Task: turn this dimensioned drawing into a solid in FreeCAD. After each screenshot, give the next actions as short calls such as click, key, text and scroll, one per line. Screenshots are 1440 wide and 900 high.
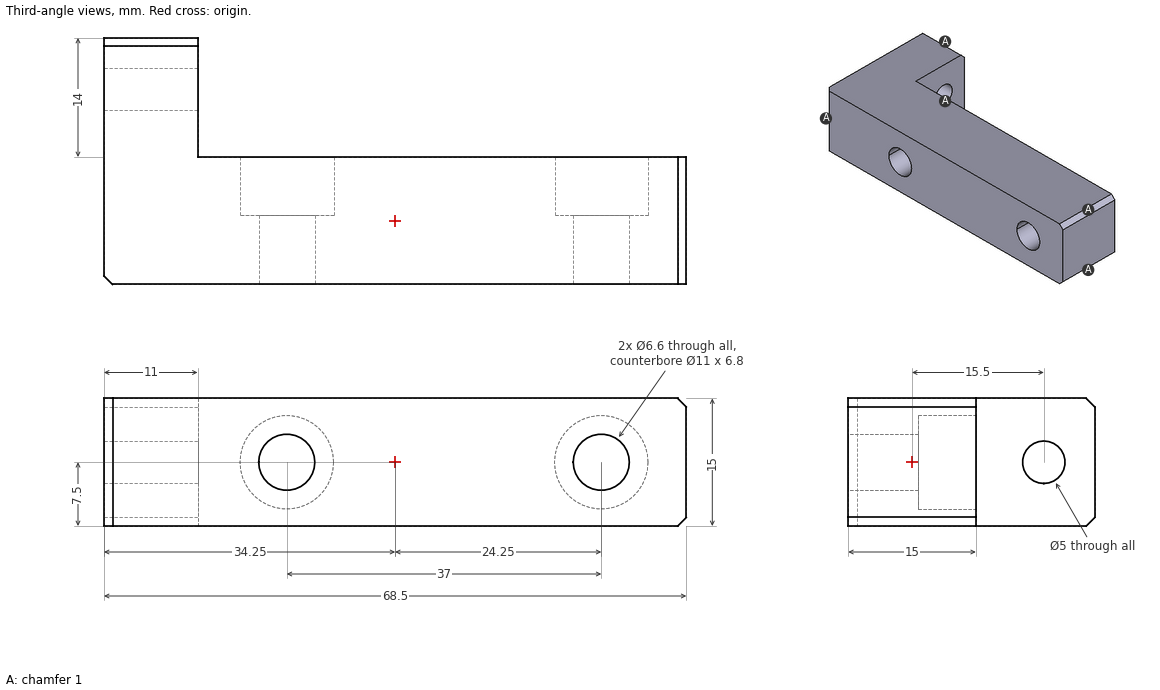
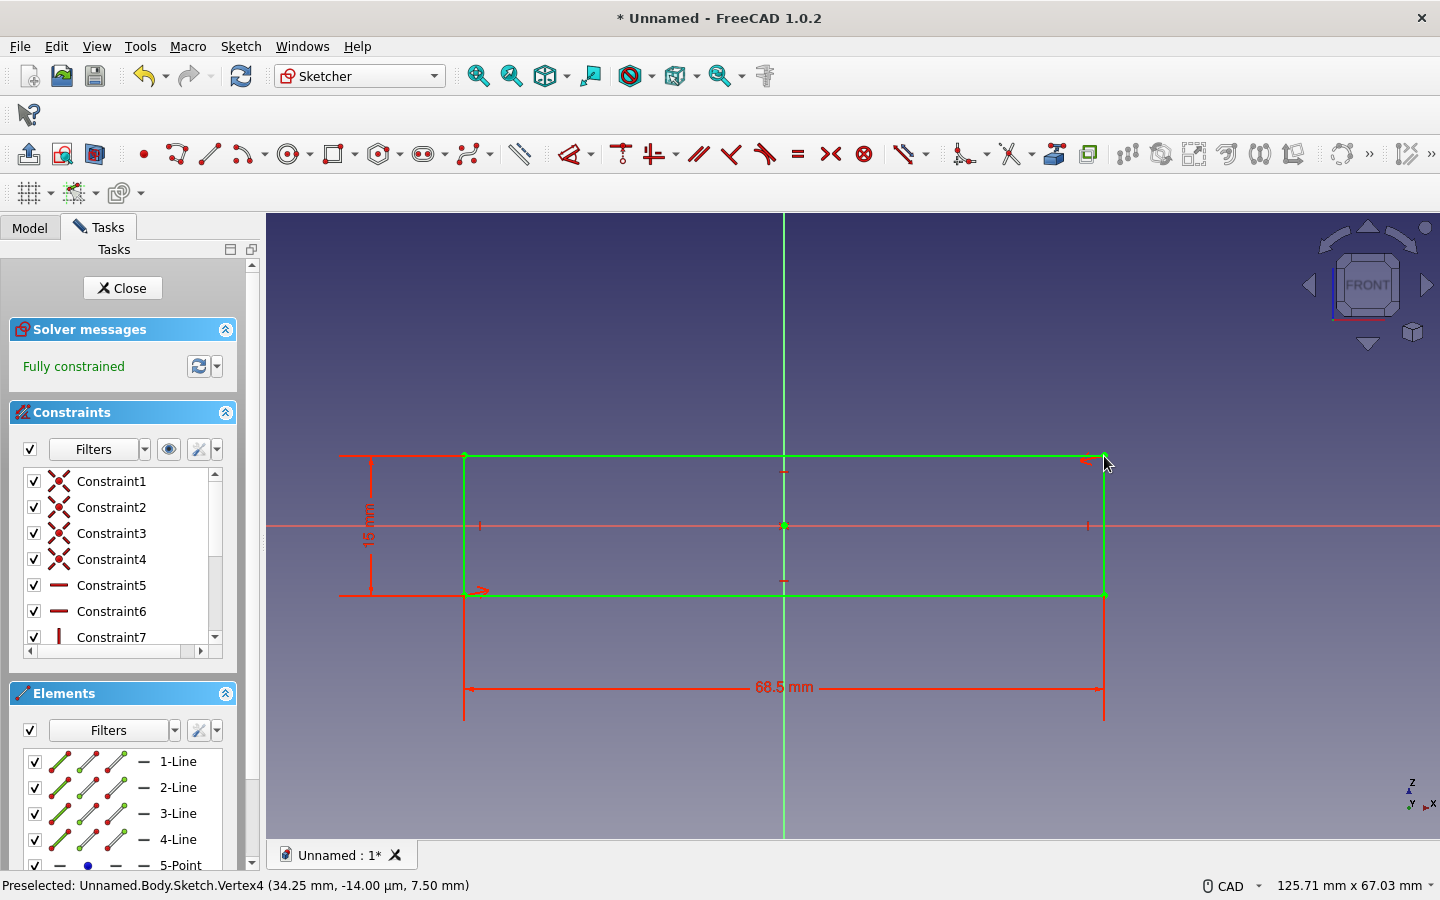
click(123, 288)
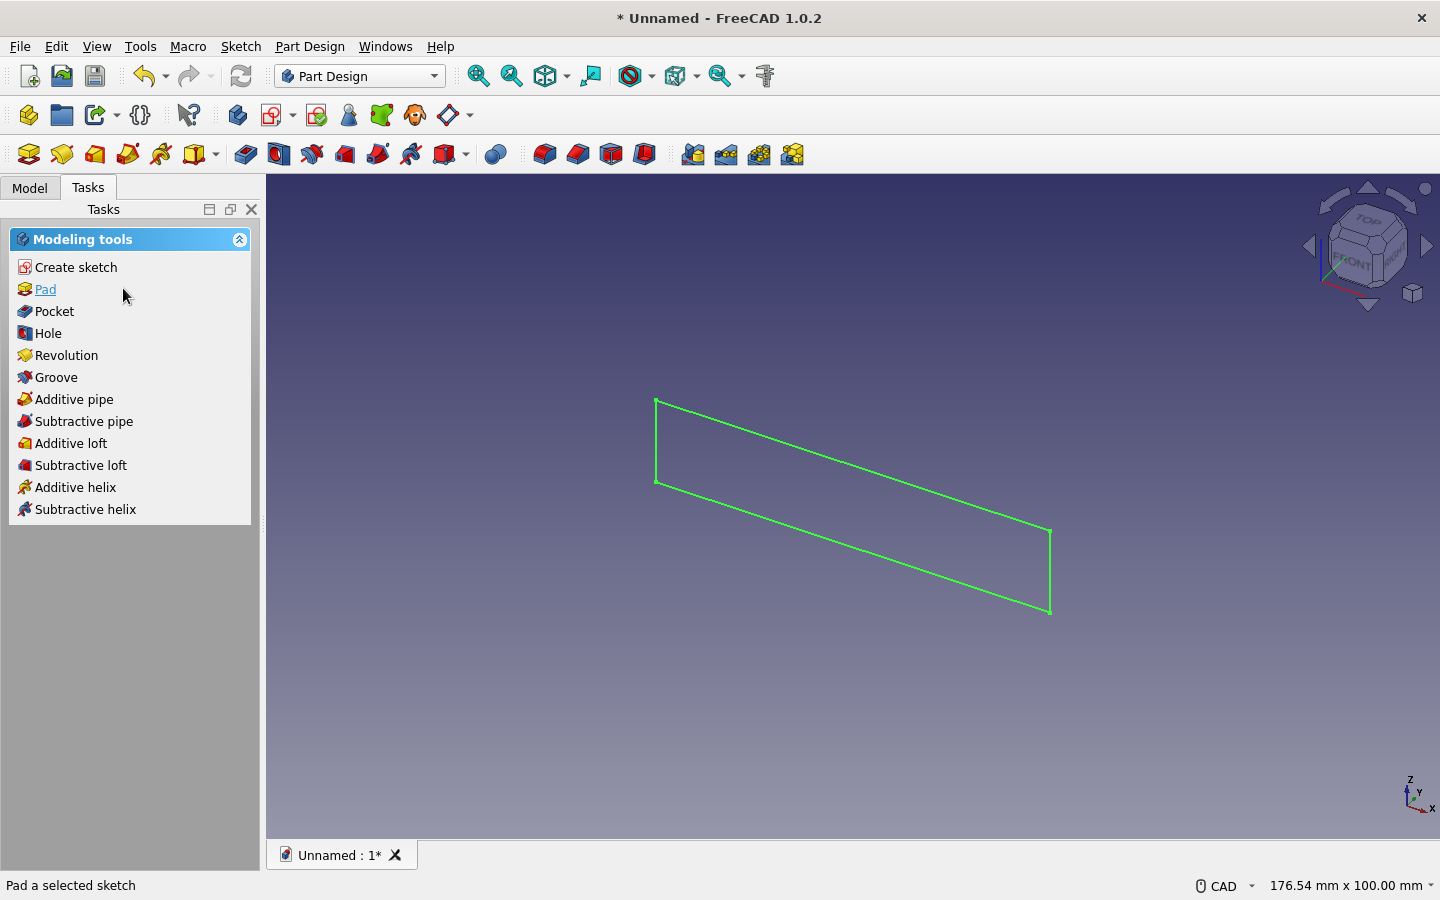
click(29, 154)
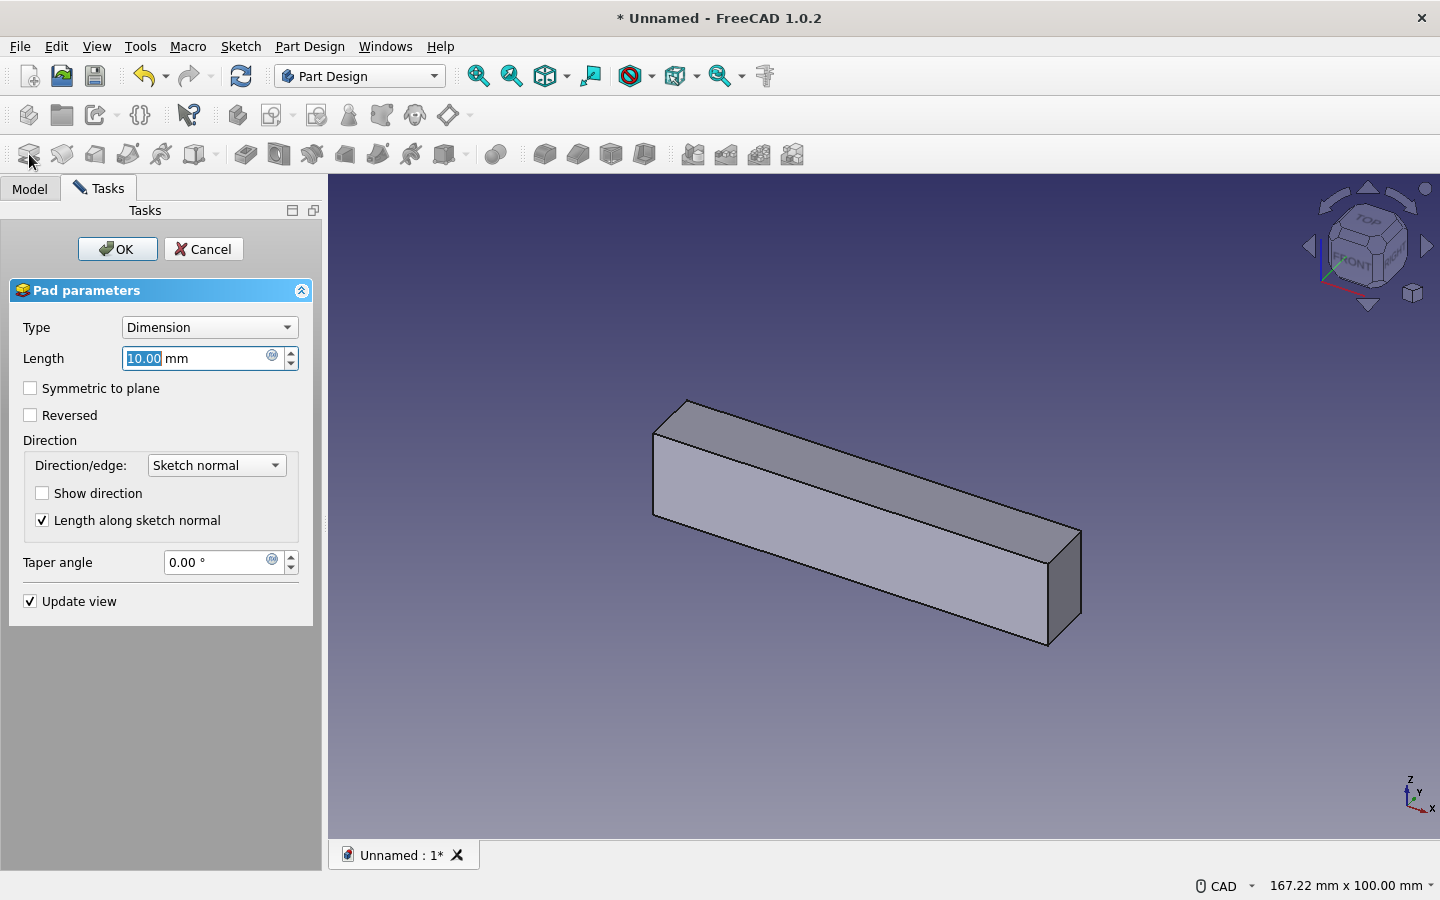
text(15)
key(Tab)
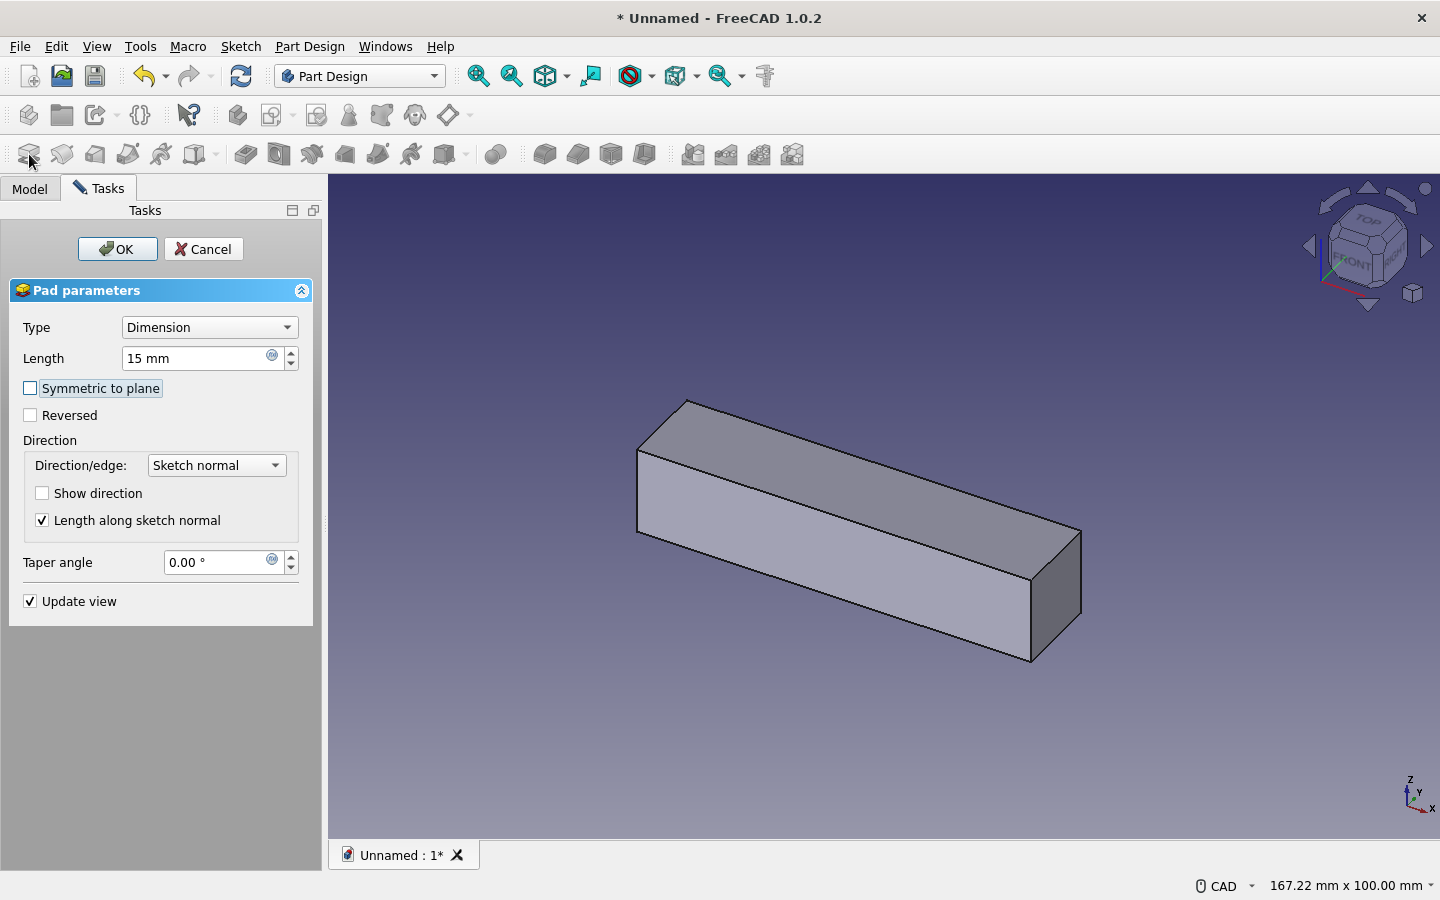
click(31, 388)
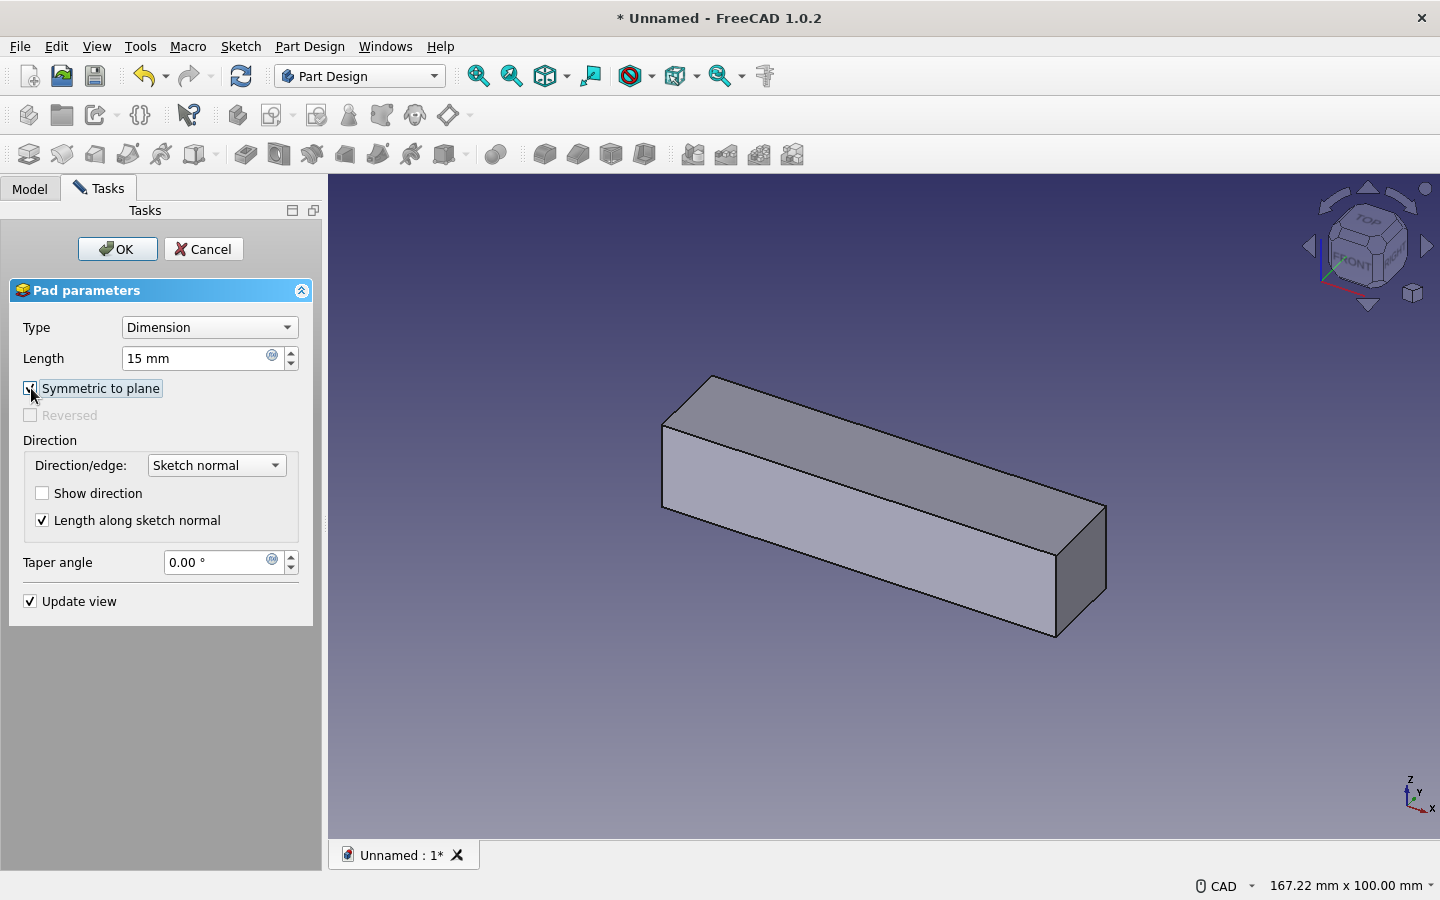
click(118, 249)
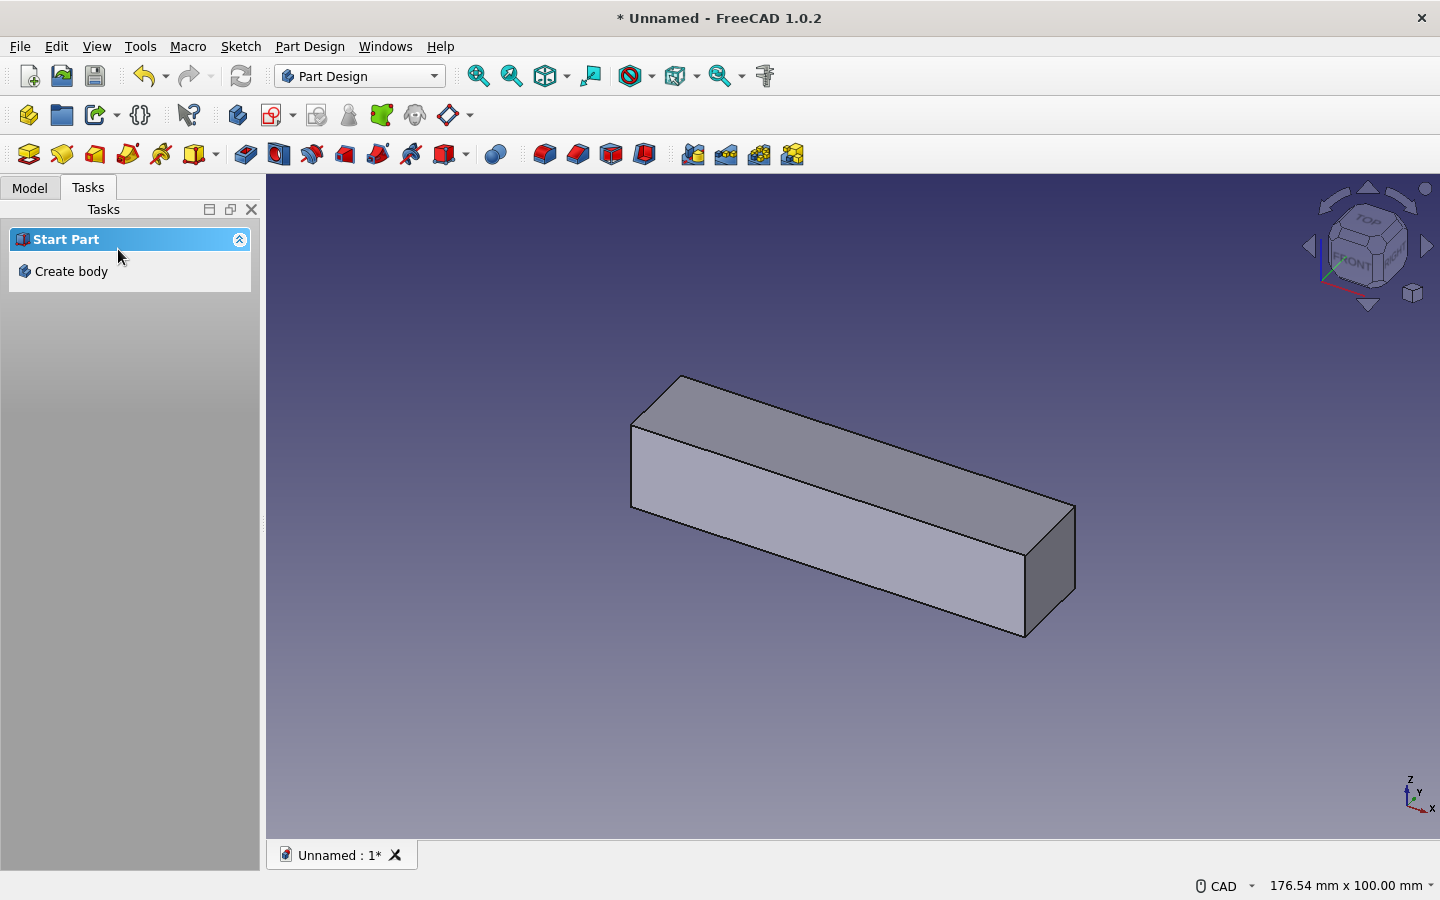
click(479, 76)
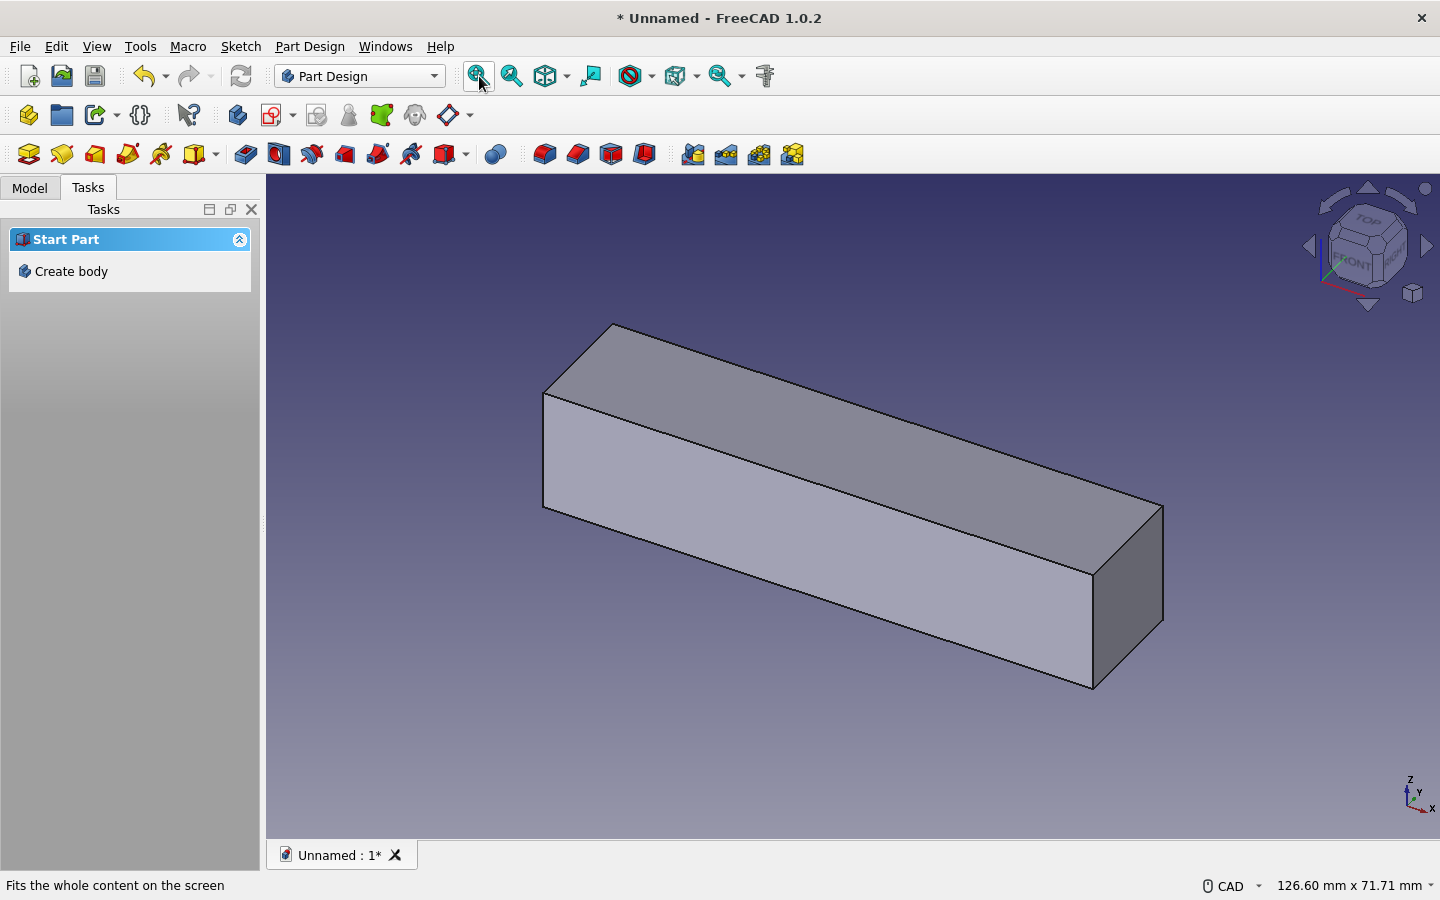
key(4)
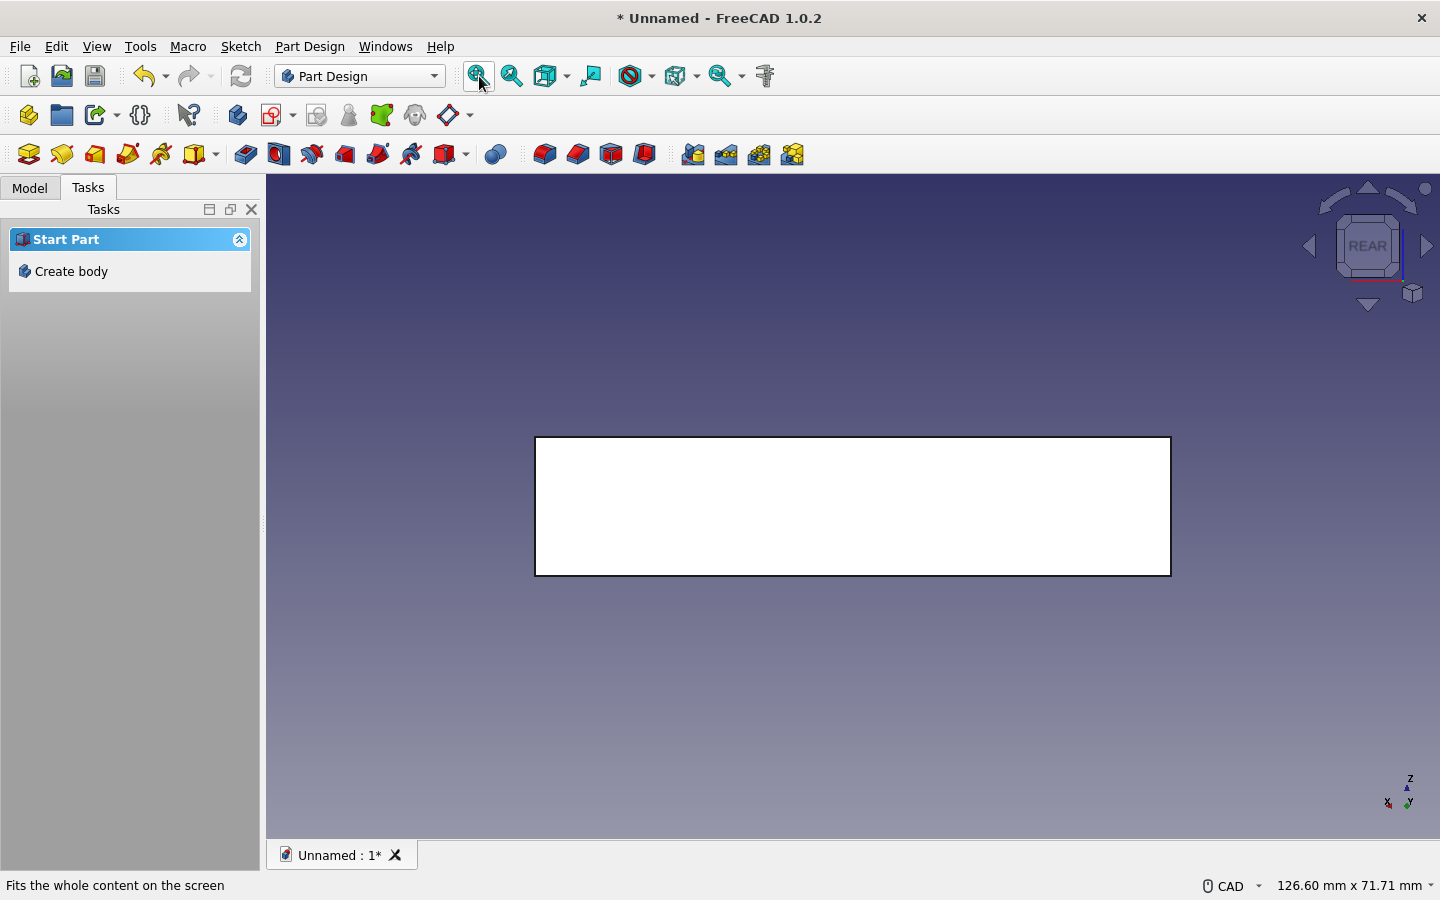
click(672, 505)